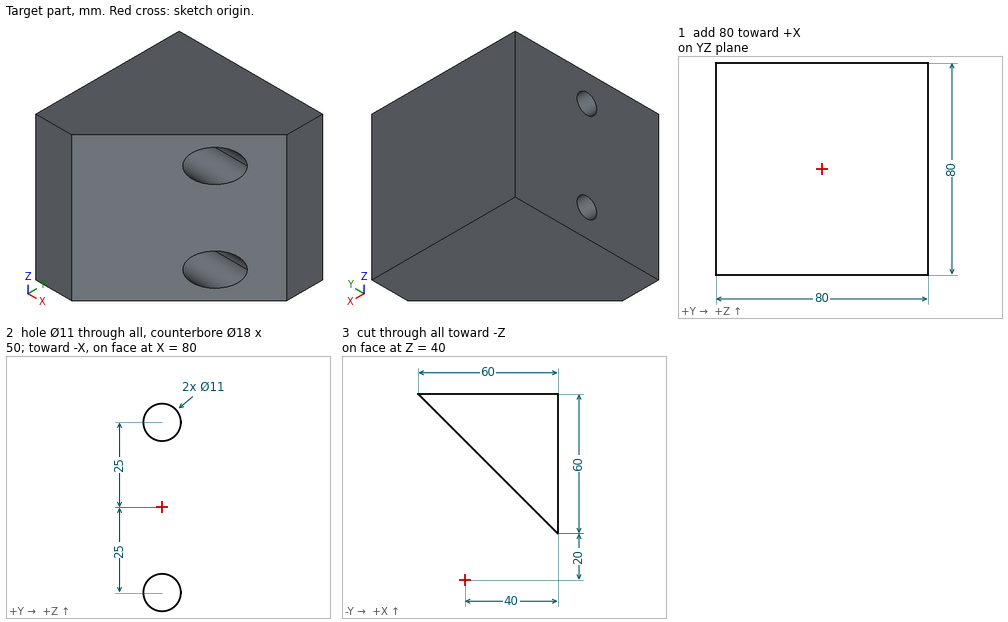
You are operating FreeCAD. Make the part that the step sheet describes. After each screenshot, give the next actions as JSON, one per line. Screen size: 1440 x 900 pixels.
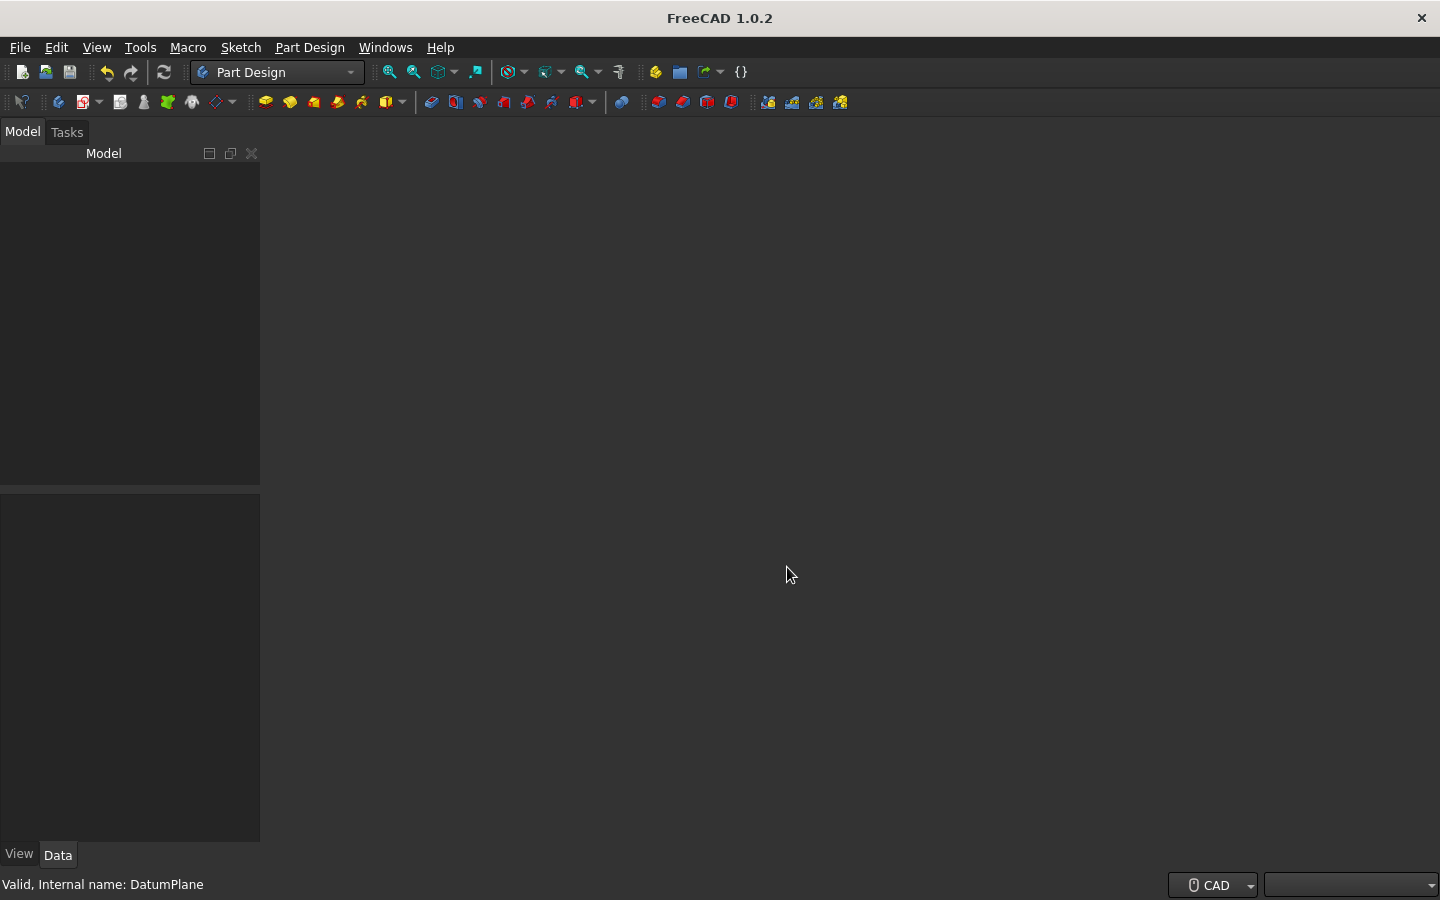
{"action": "key", "text": "ctrl+n"}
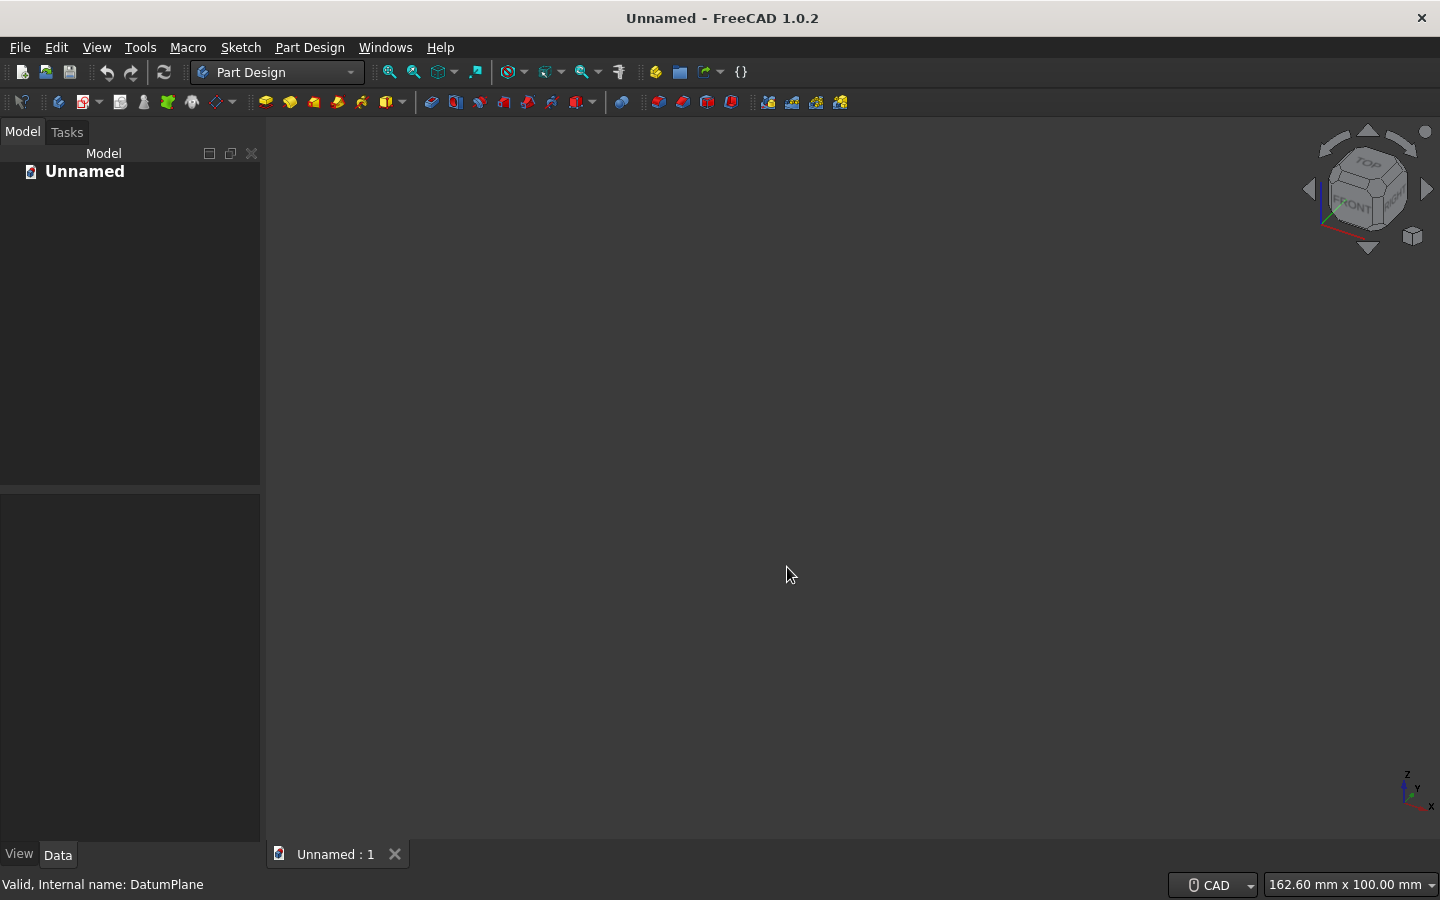
{"action": "left_click", "coordinate": [84, 102]}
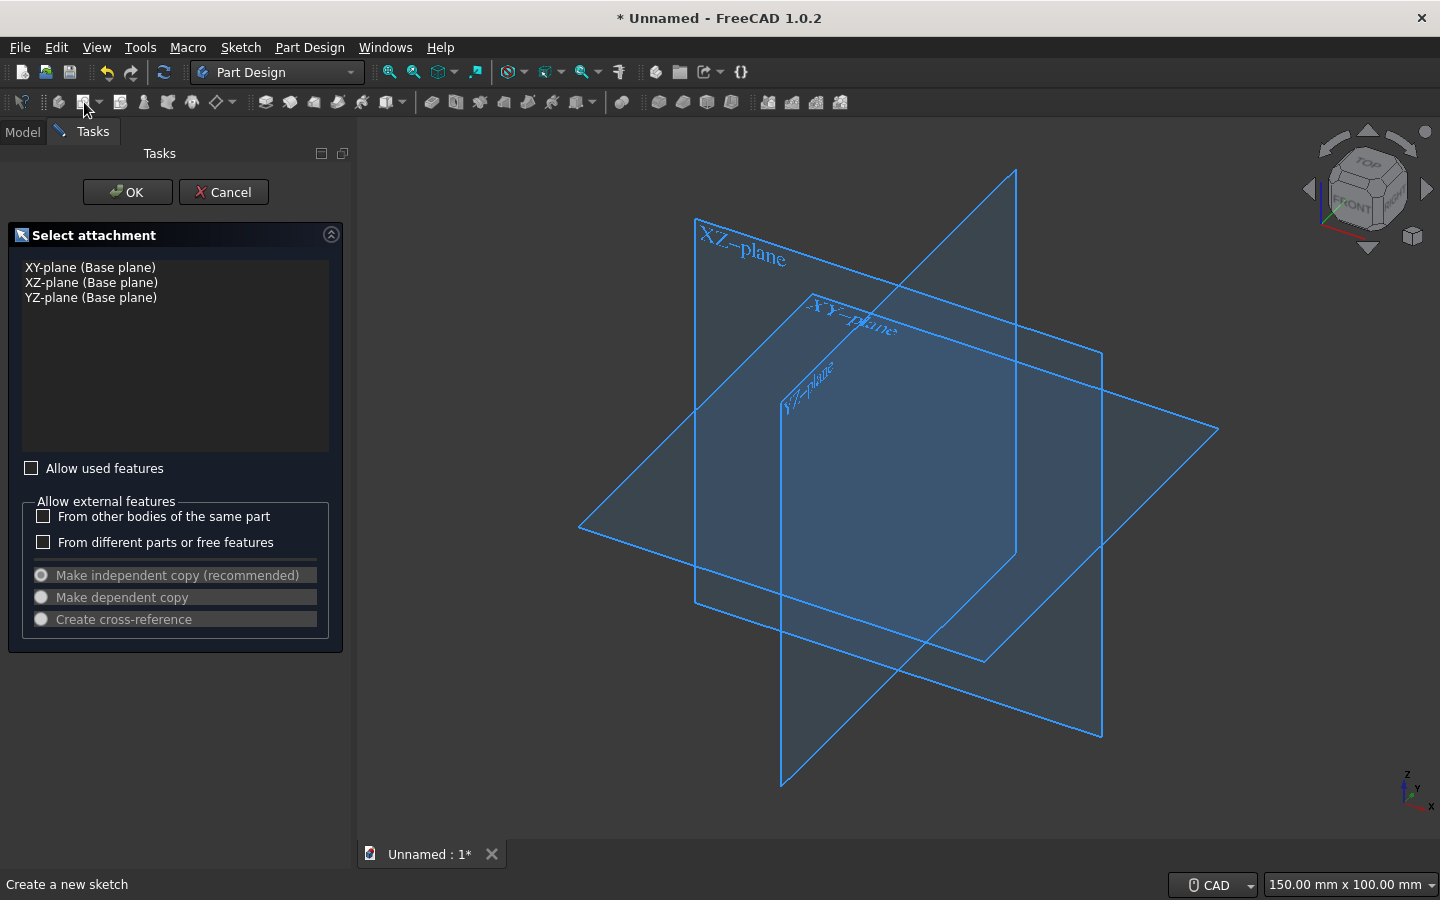
{"action": "left_click", "coordinate": [82, 298]}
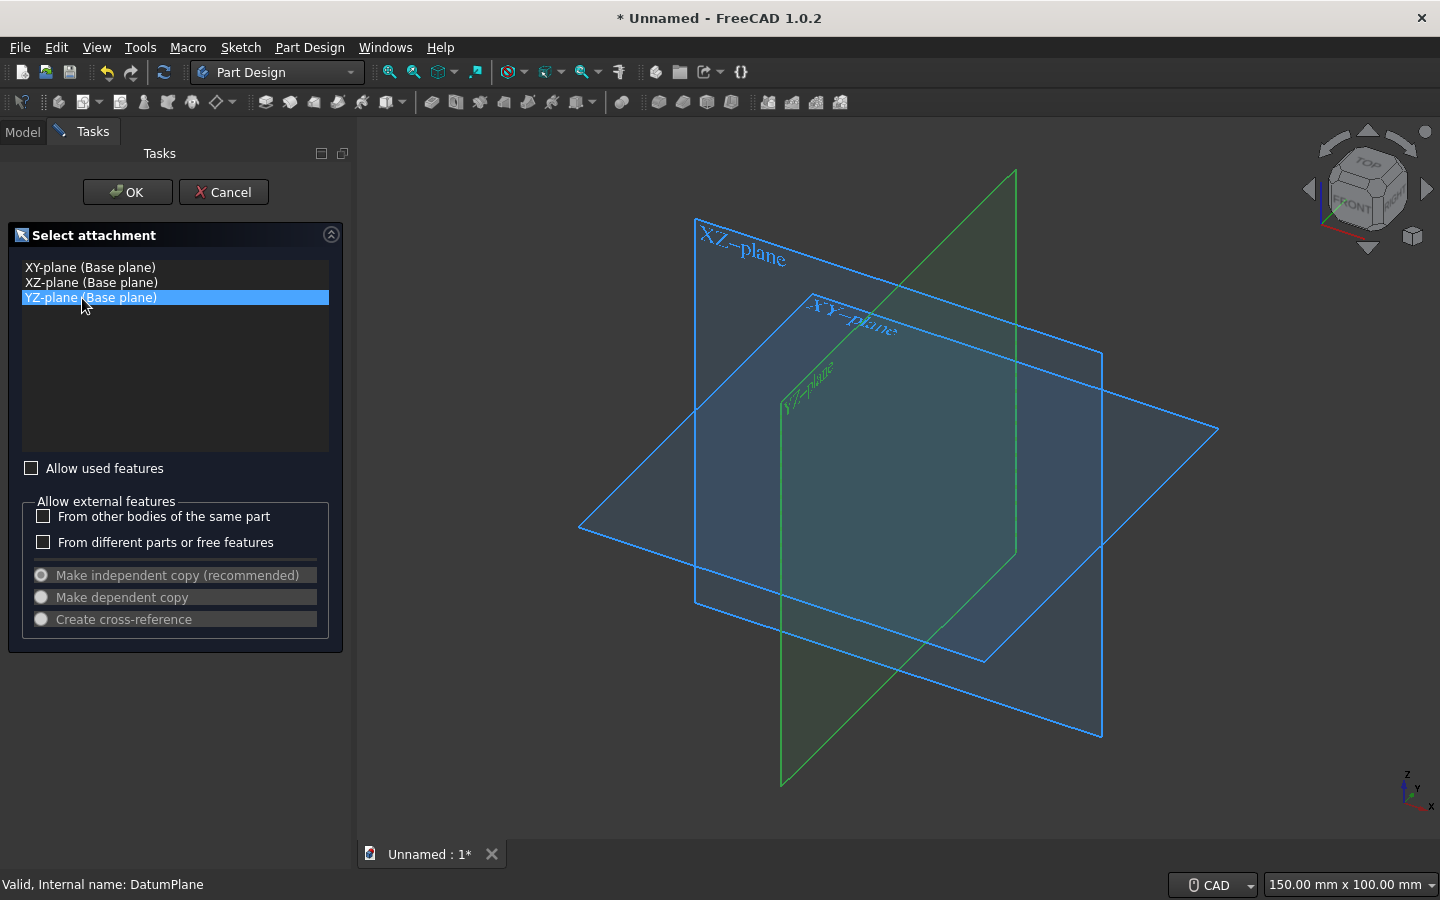
{"action": "left_click", "coordinate": [128, 192]}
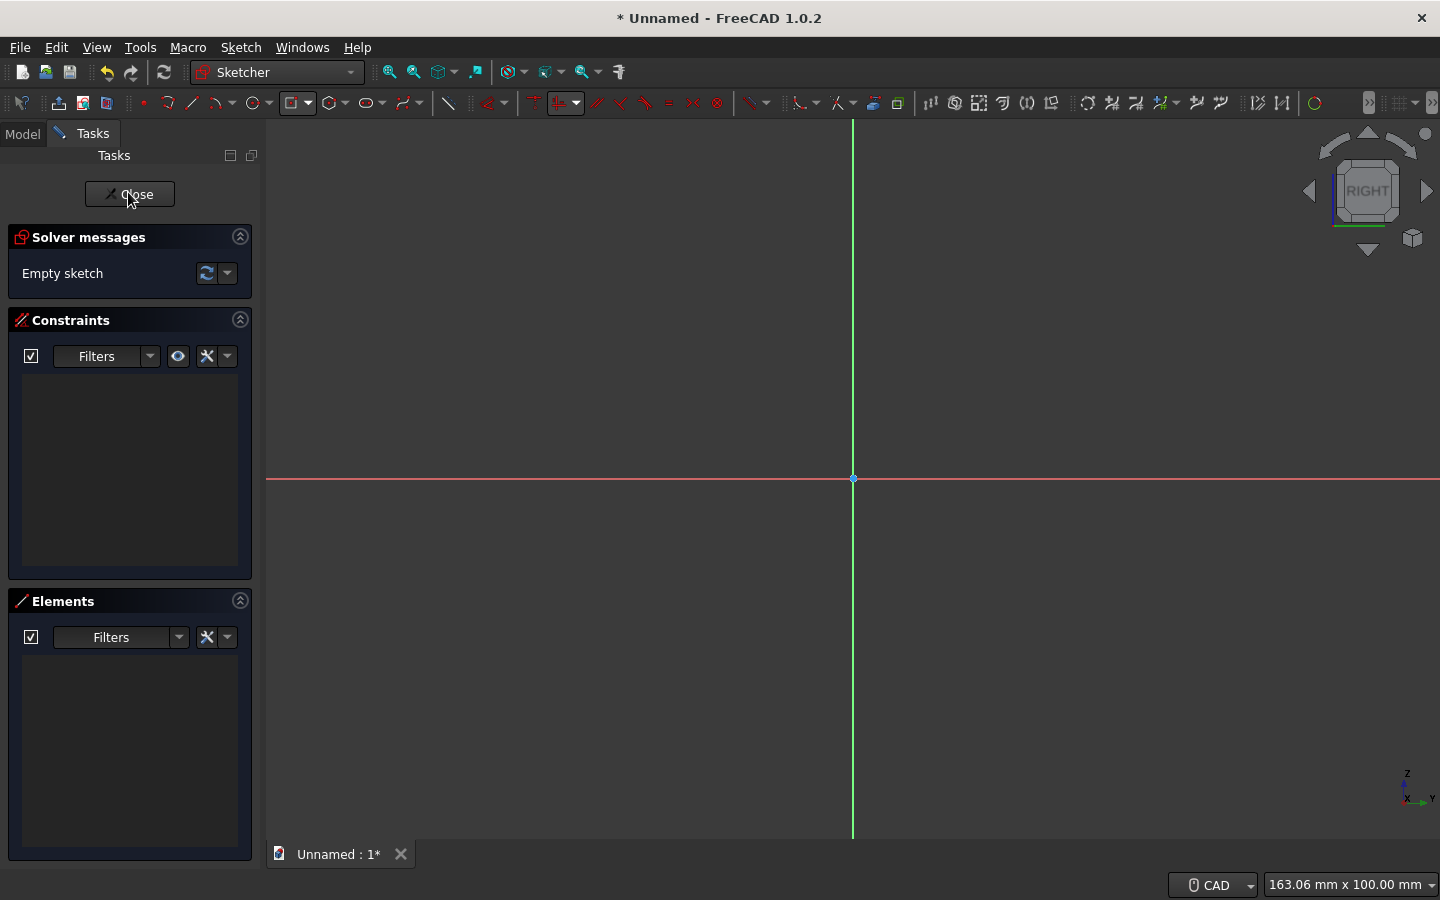
{"action": "left_click", "coordinate": [292, 104]}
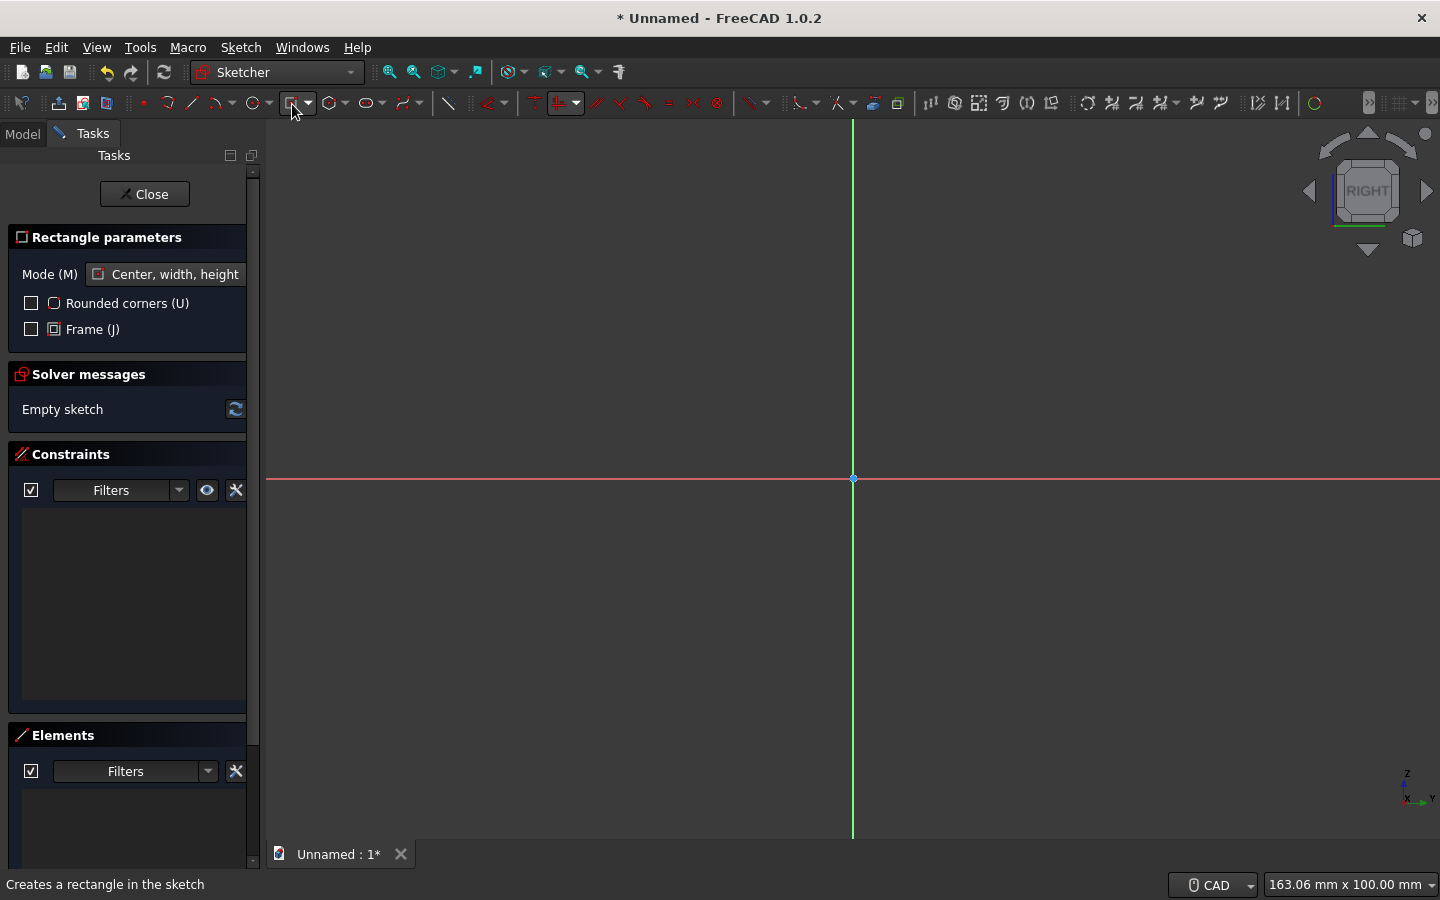
{"action": "left_click", "coordinate": [853, 479]}
{"action": "left_click", "coordinate": [1141, 191]}
{"action": "key", "text": "Escape"}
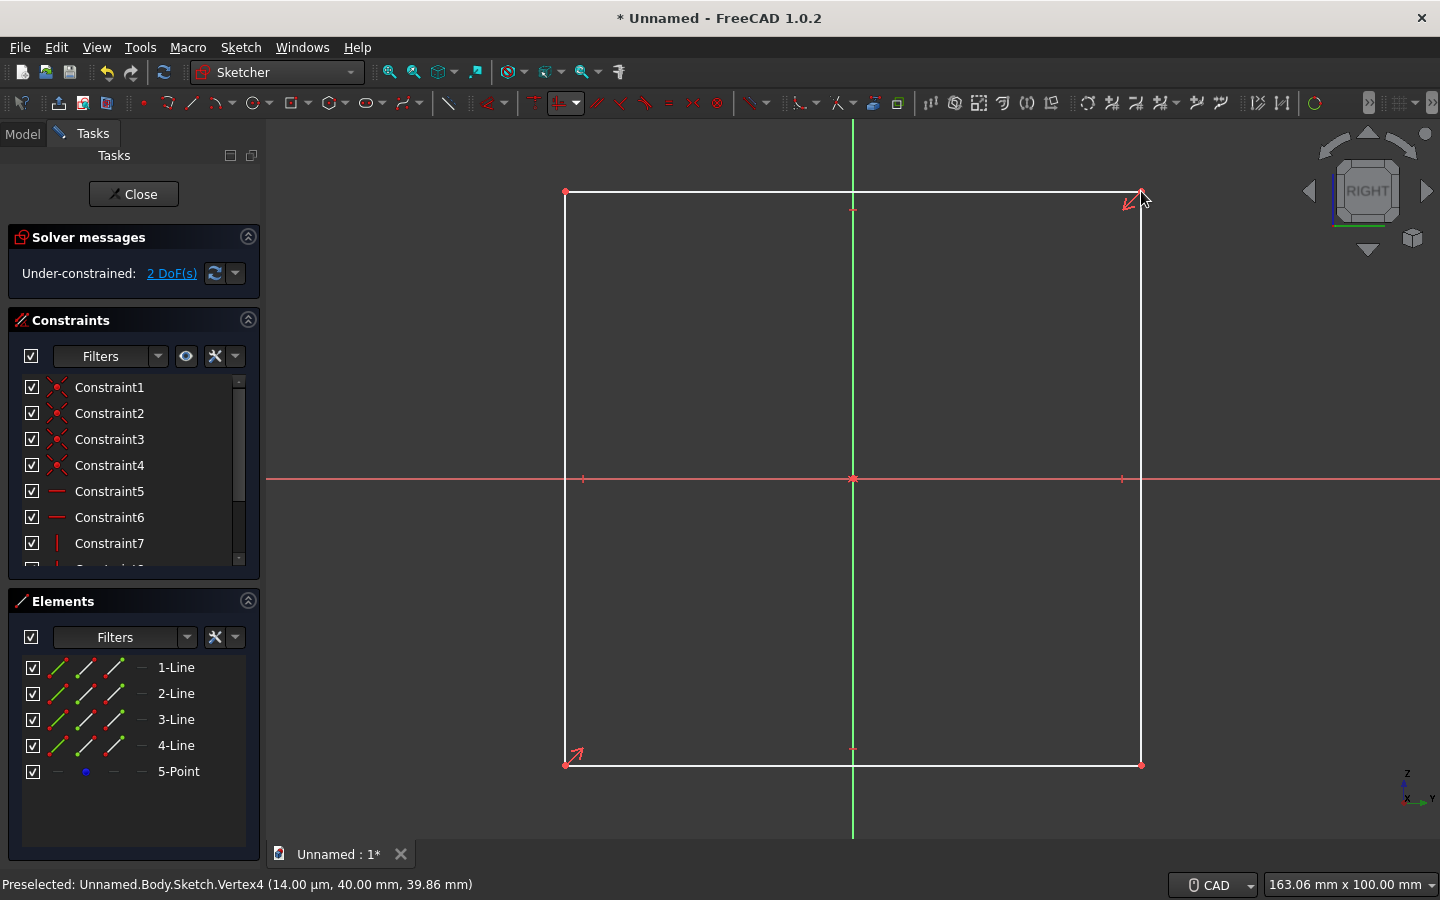
{"action": "key", "text": "d"}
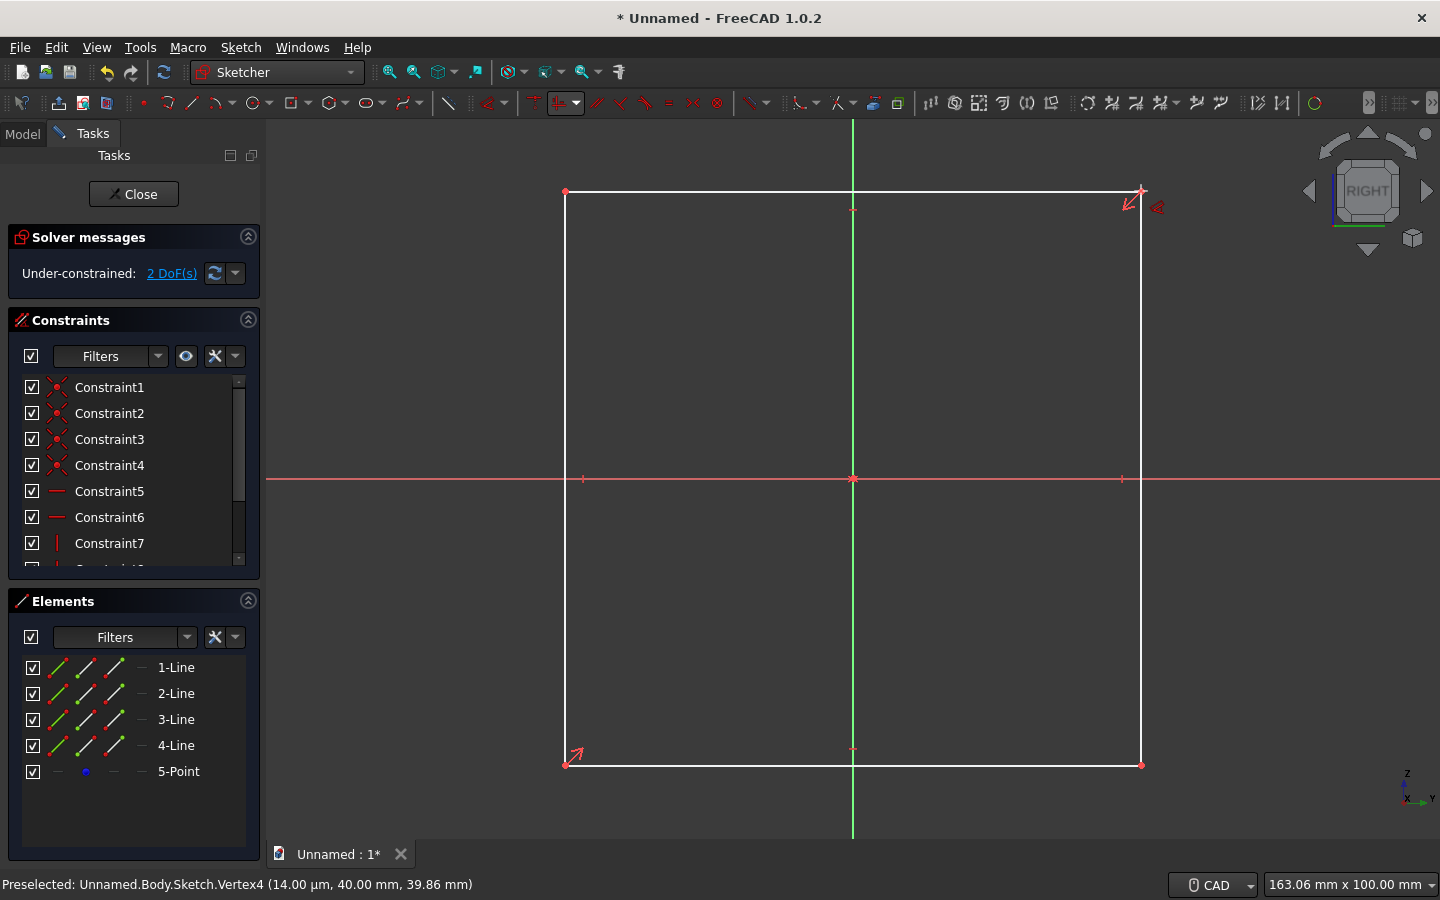
{"action": "left_click", "coordinate": [738, 766]}
{"action": "left_click", "coordinate": [721, 800]}